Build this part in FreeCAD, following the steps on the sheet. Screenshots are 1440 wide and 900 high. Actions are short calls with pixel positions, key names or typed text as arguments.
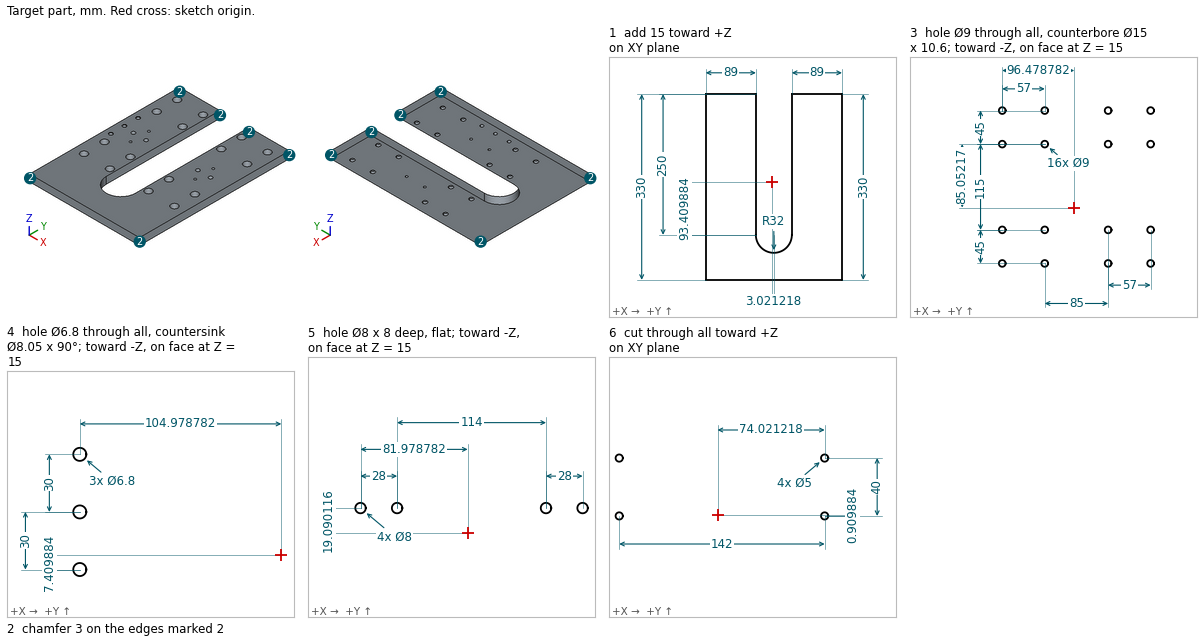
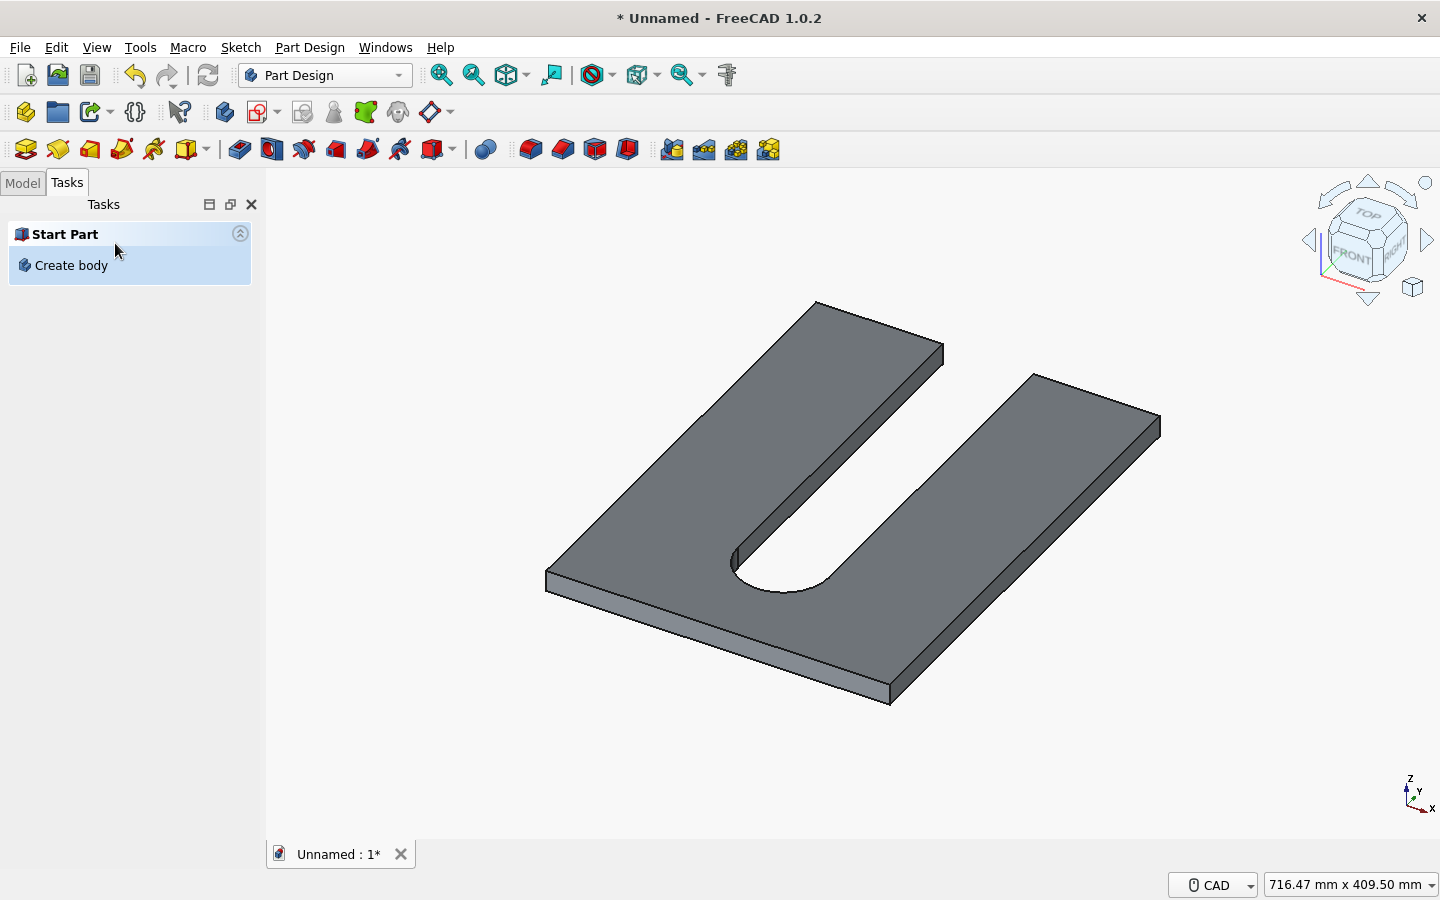
click(890, 694)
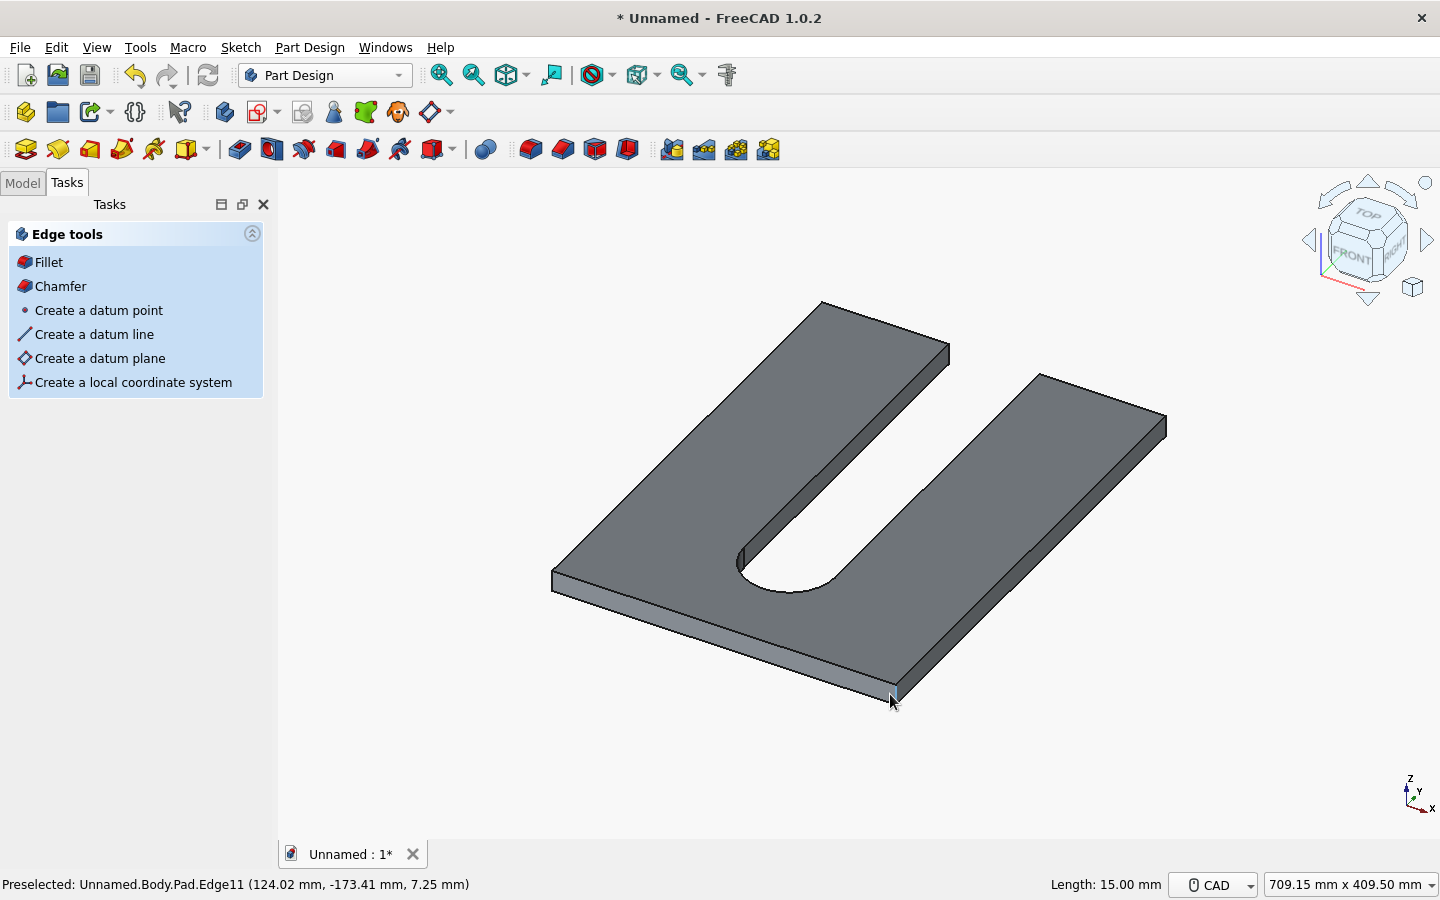
key(0)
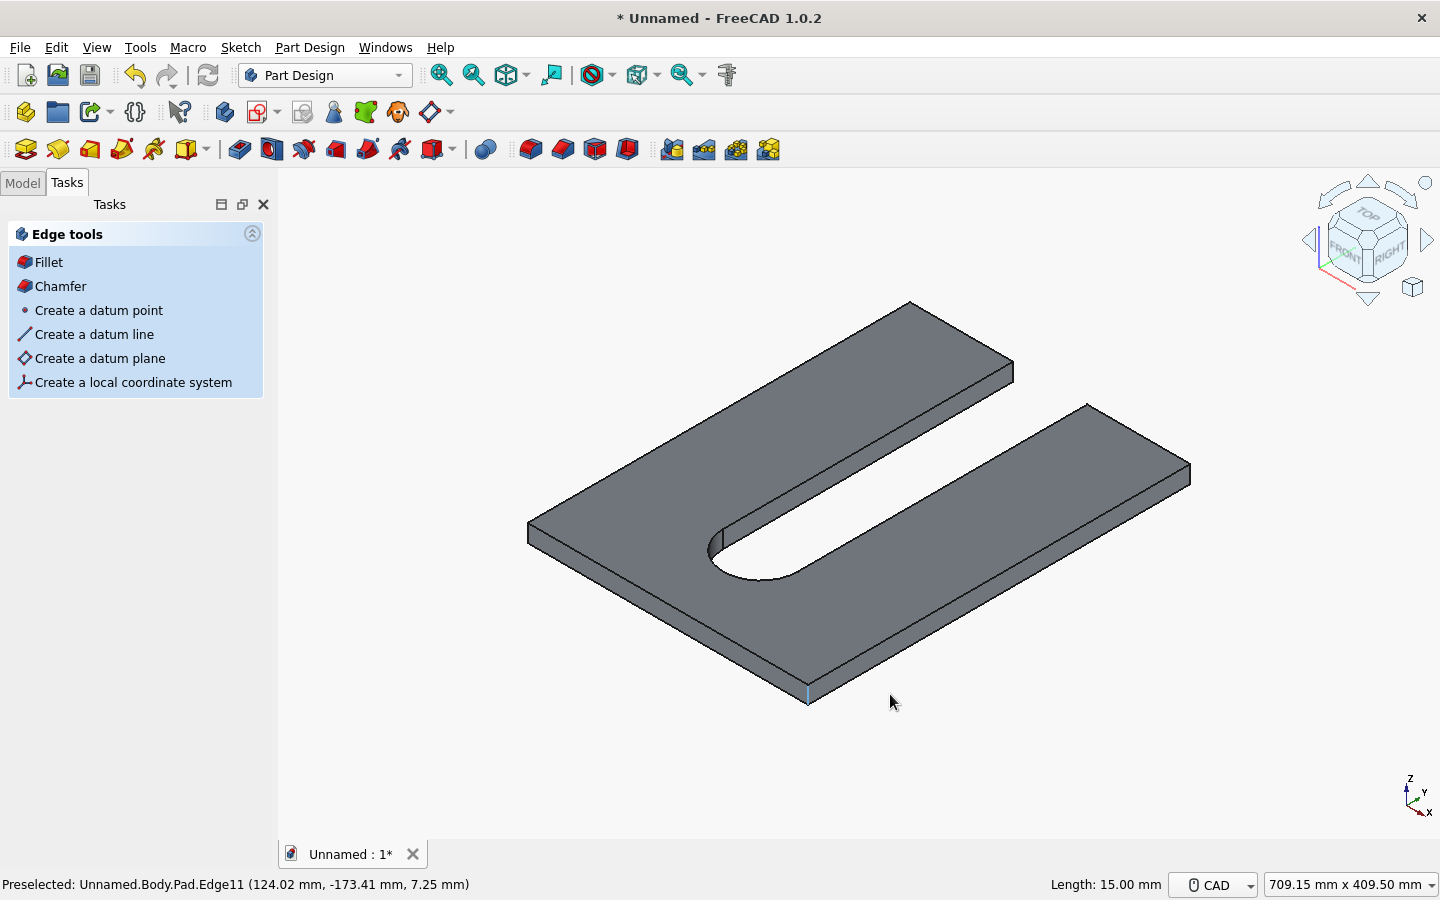
key(2)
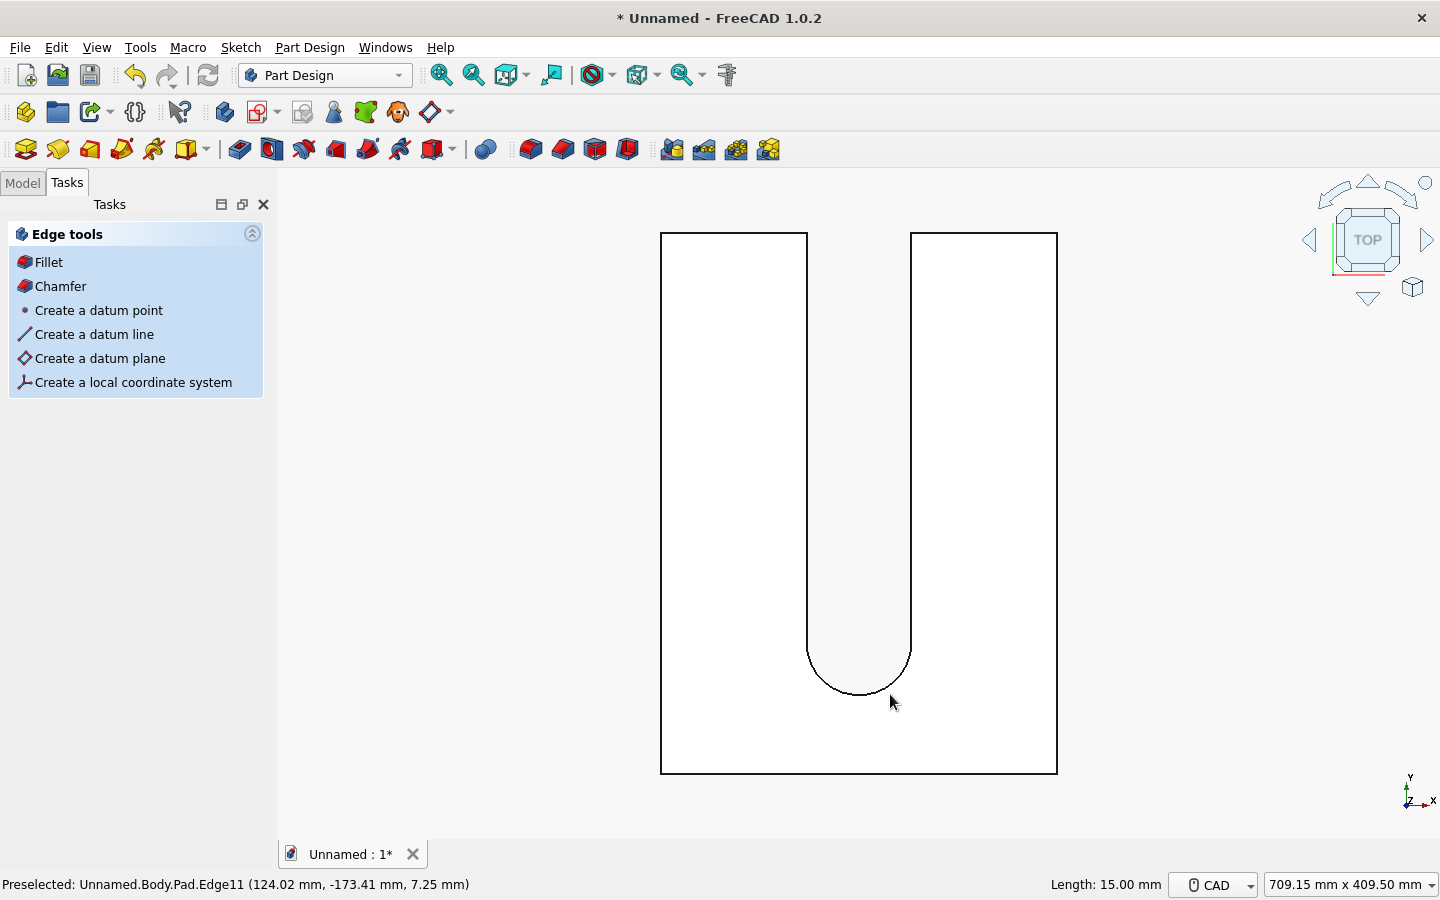
key(1)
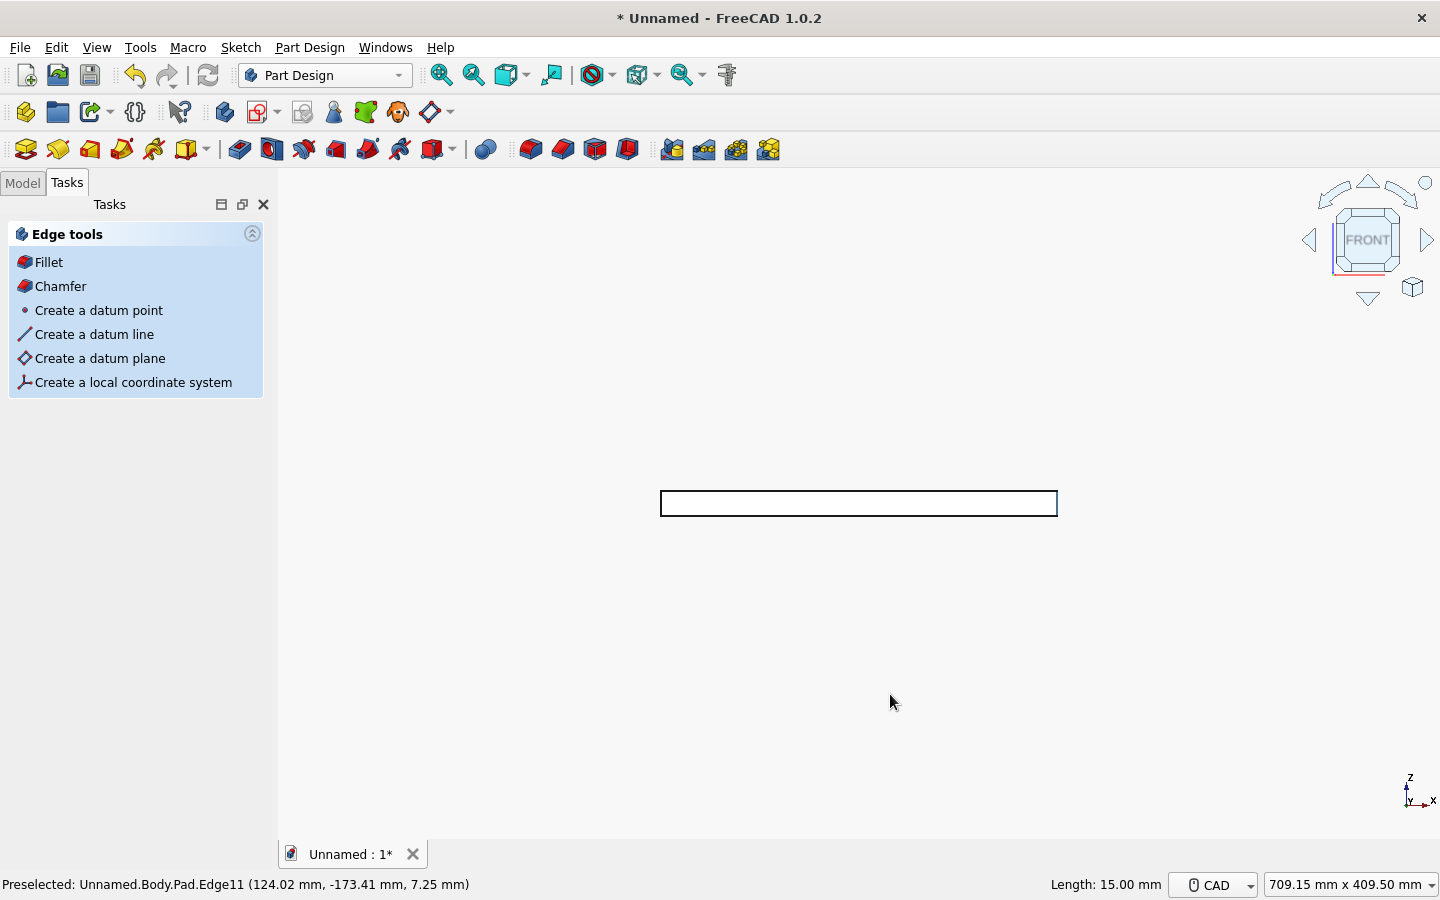
key(v)
key(f)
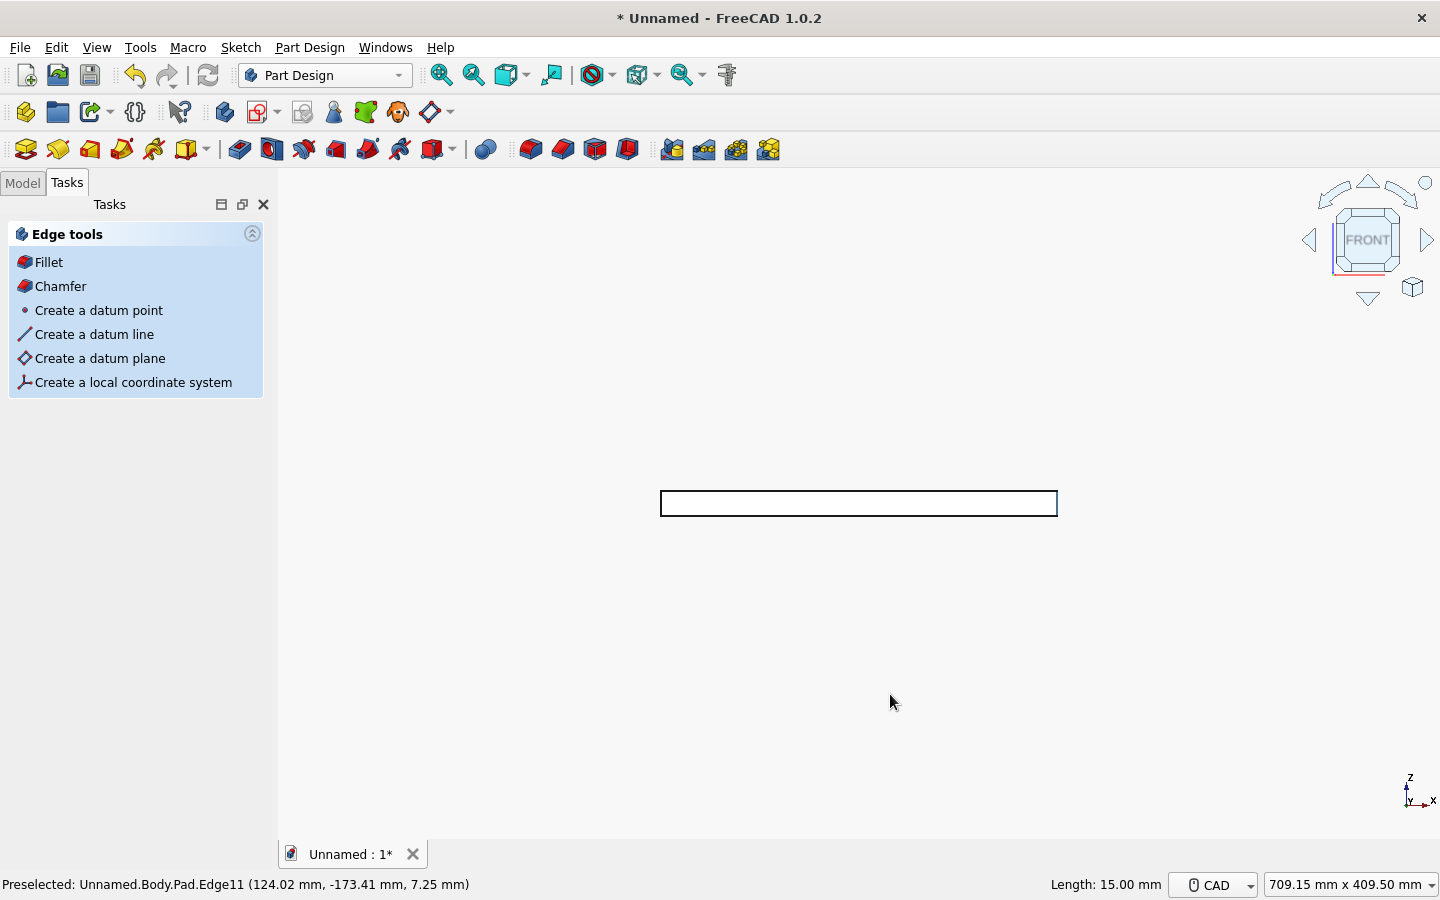
click(661, 503, ctrl)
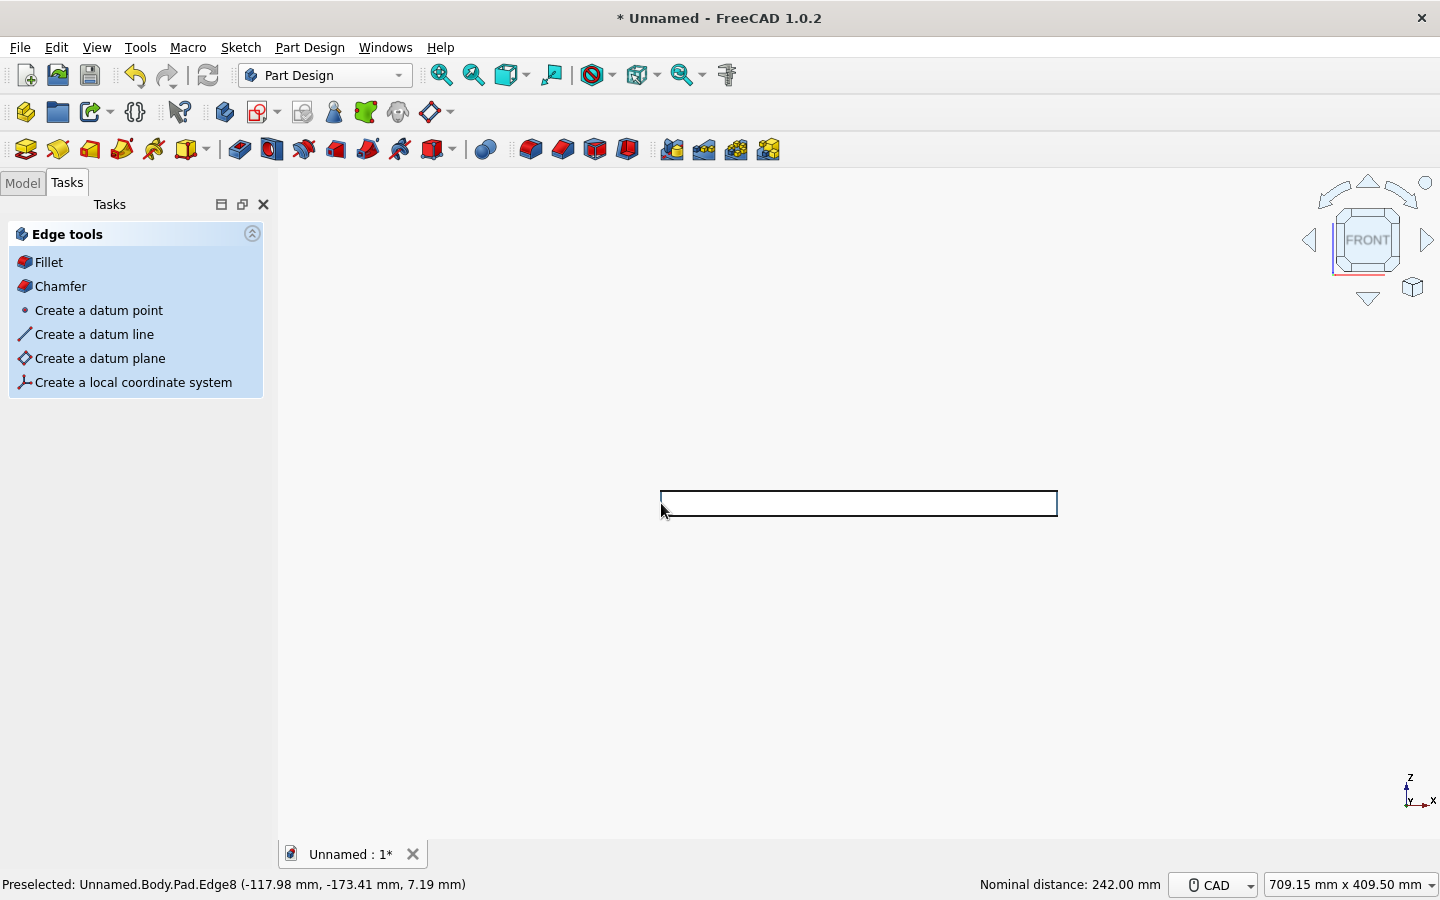
key(3)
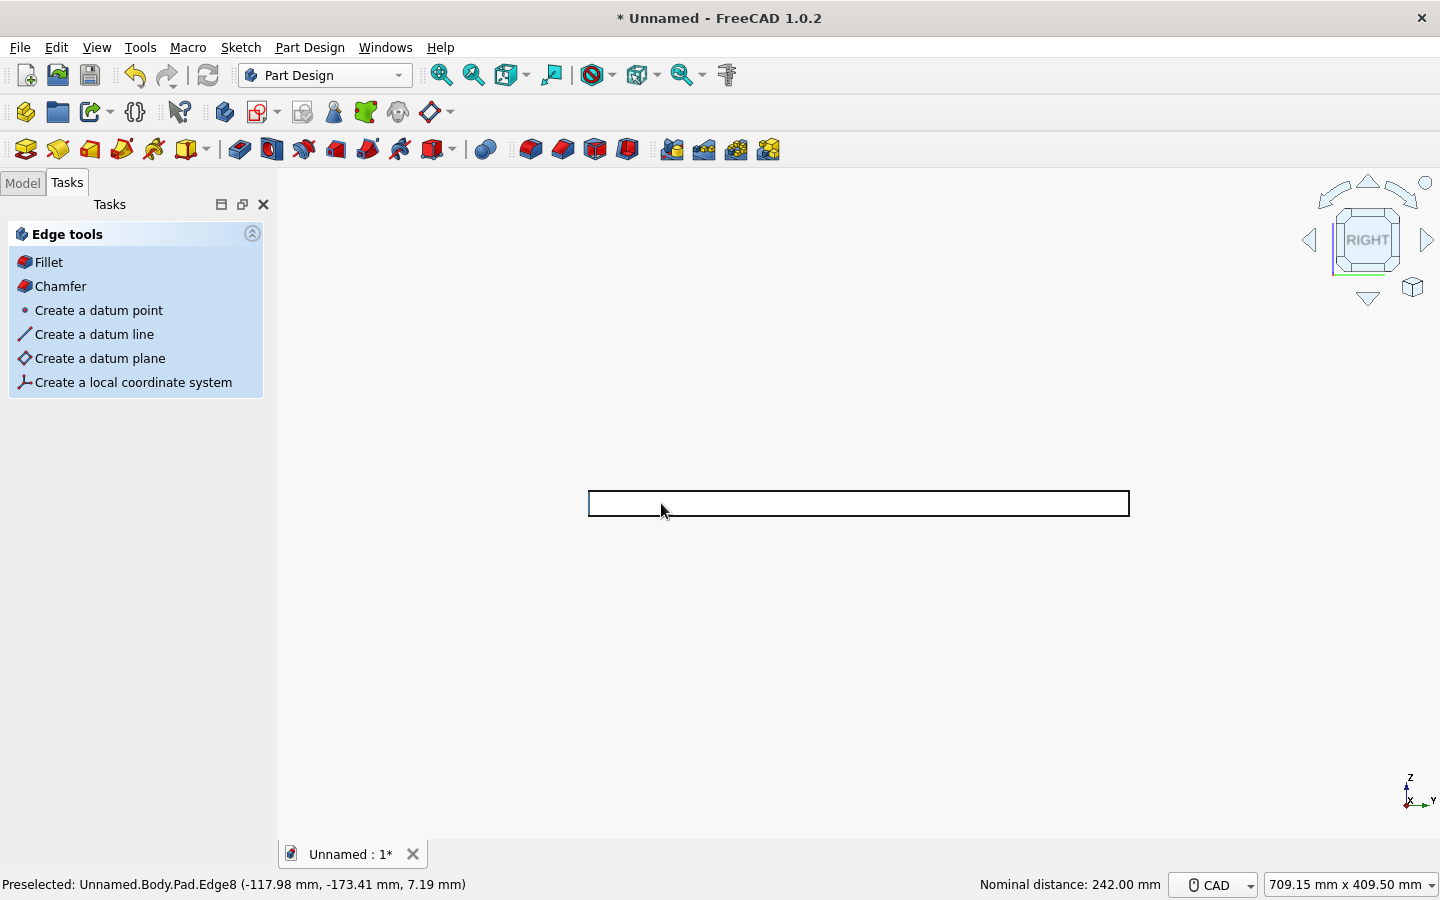
click(1129, 502, ctrl)